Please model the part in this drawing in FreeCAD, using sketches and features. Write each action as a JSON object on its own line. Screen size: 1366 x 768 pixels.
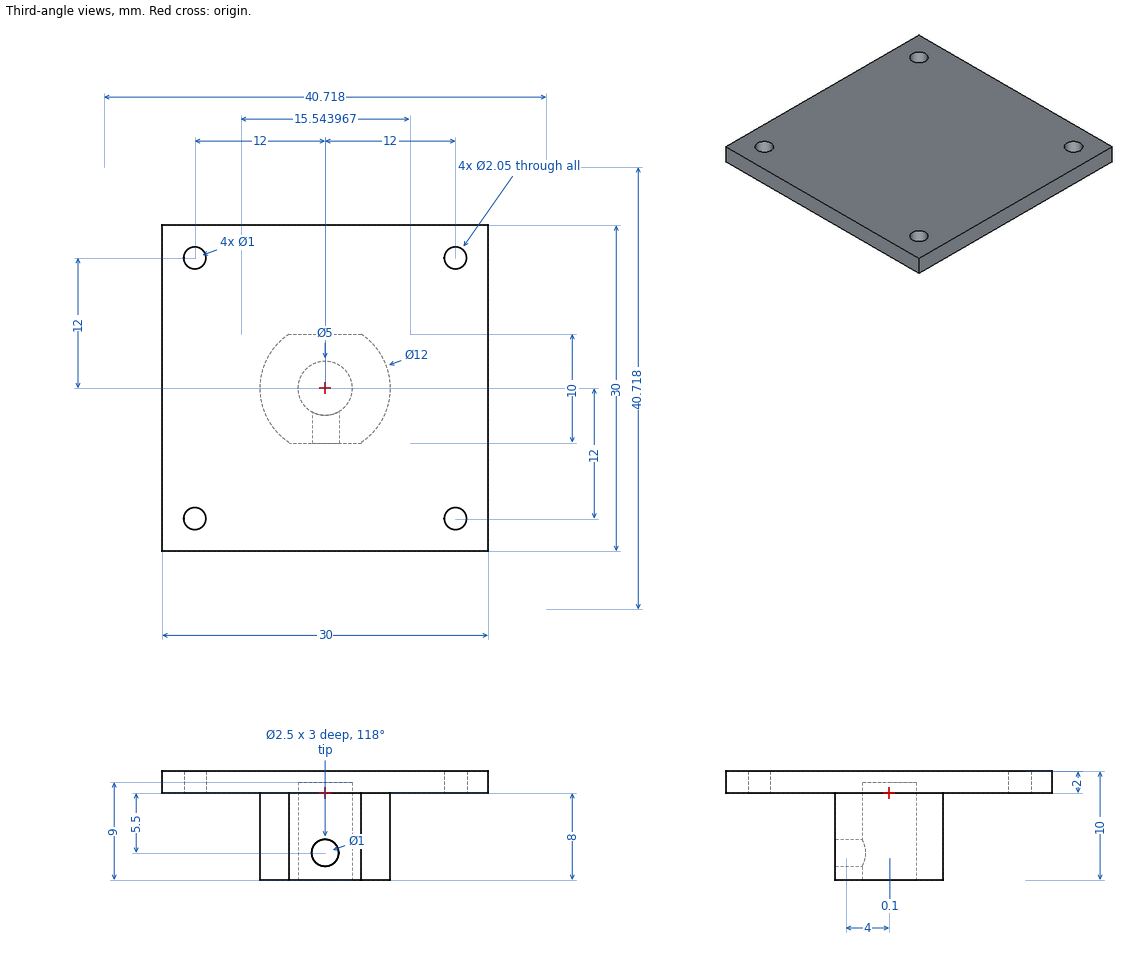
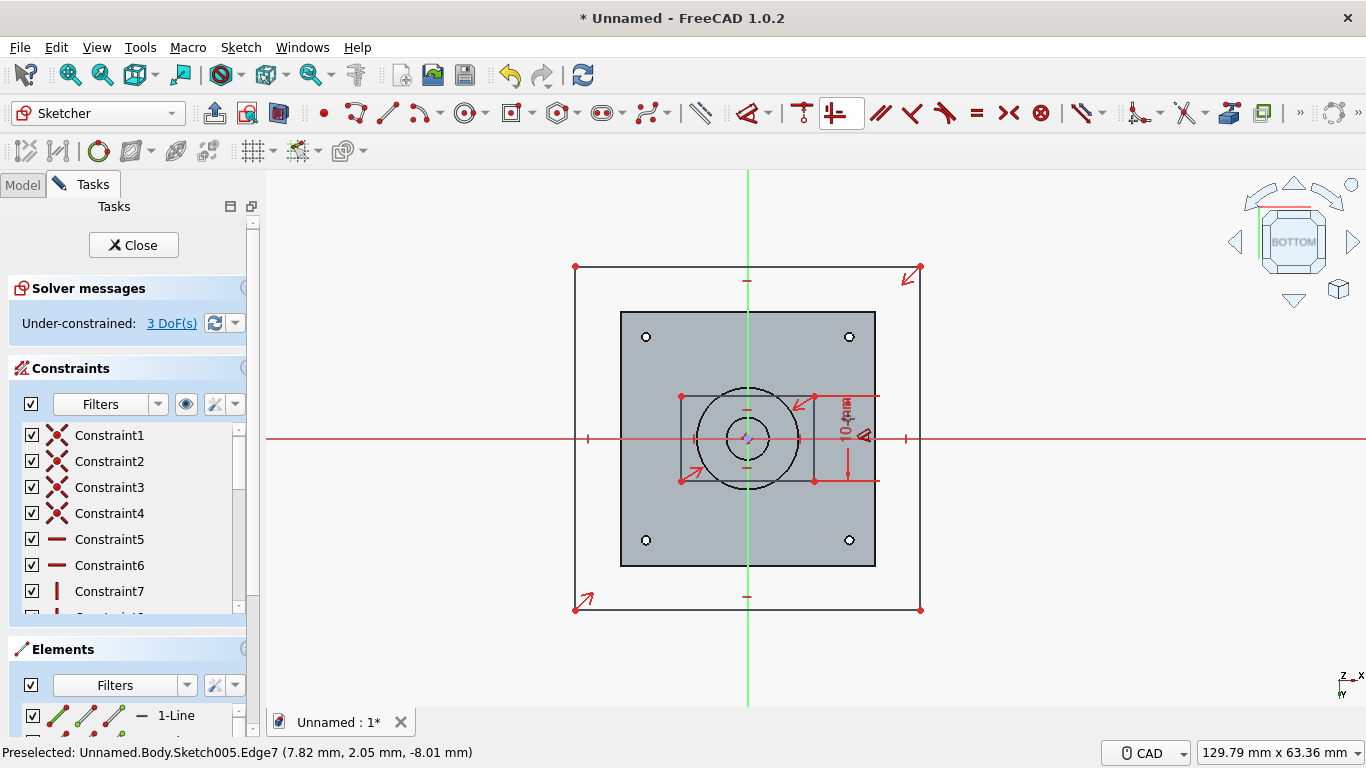
{"action": "left_click", "coordinate": [679, 610]}
{"action": "left_click", "coordinate": [668, 644]}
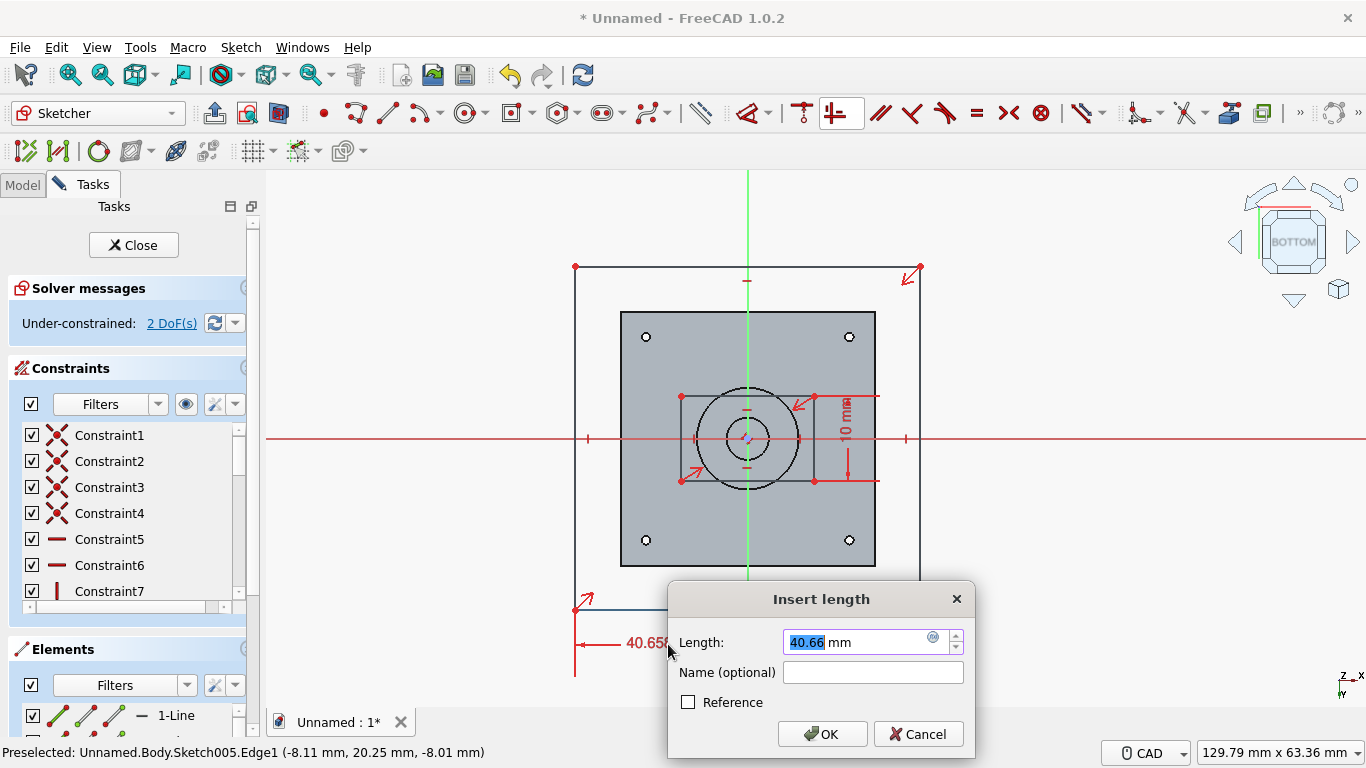
{"action": "type", "text": "40.718"}
{"action": "key", "text": "Return"}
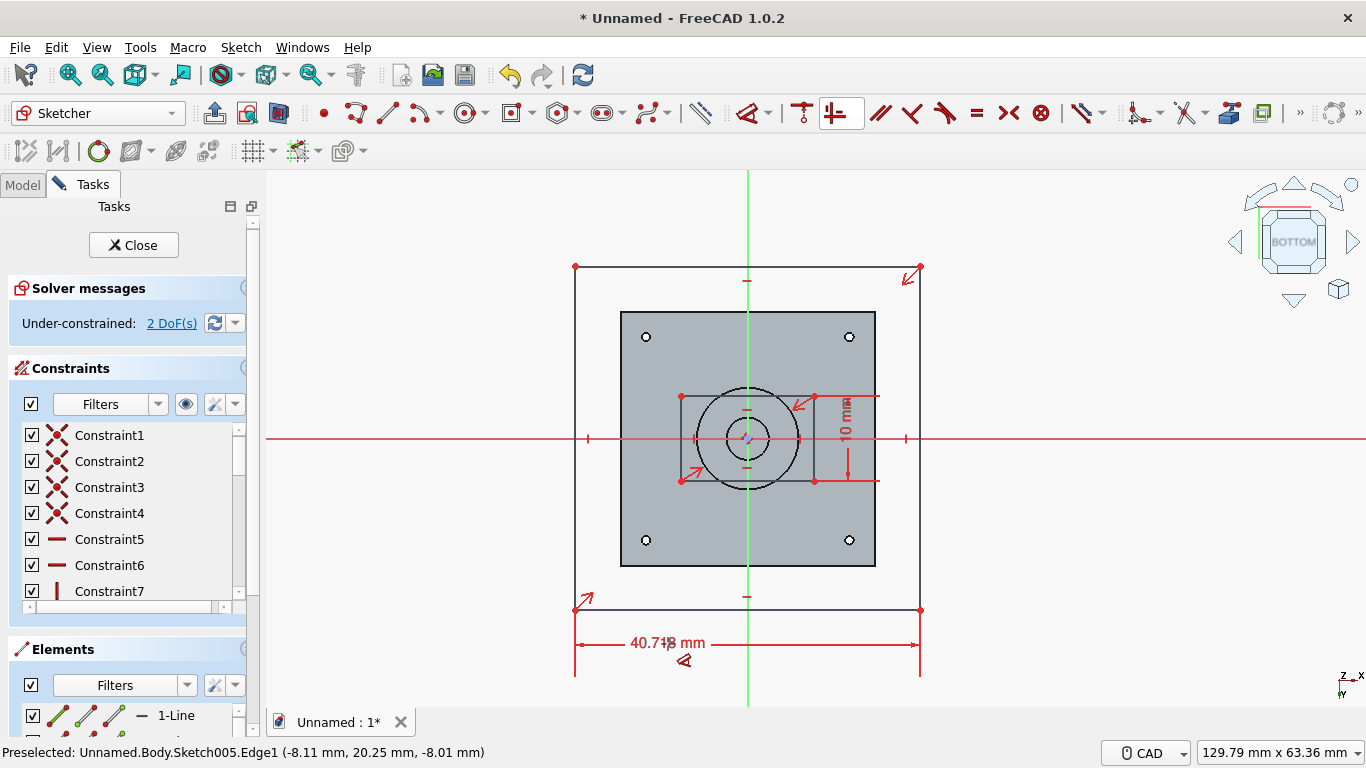
{"action": "left_click", "coordinate": [920, 507]}
{"action": "left_click", "coordinate": [954, 360]}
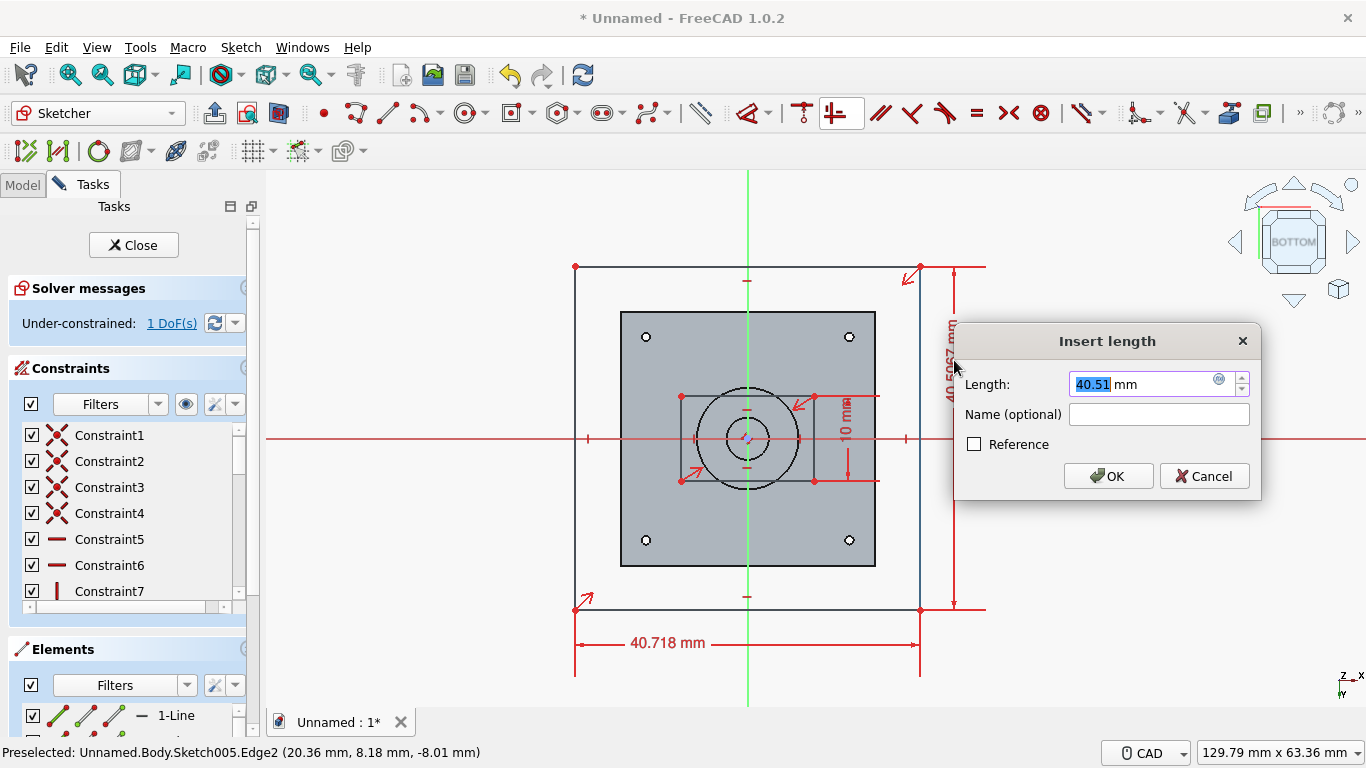
{"action": "type", "text": "40.718"}
{"action": "key", "text": "Return"}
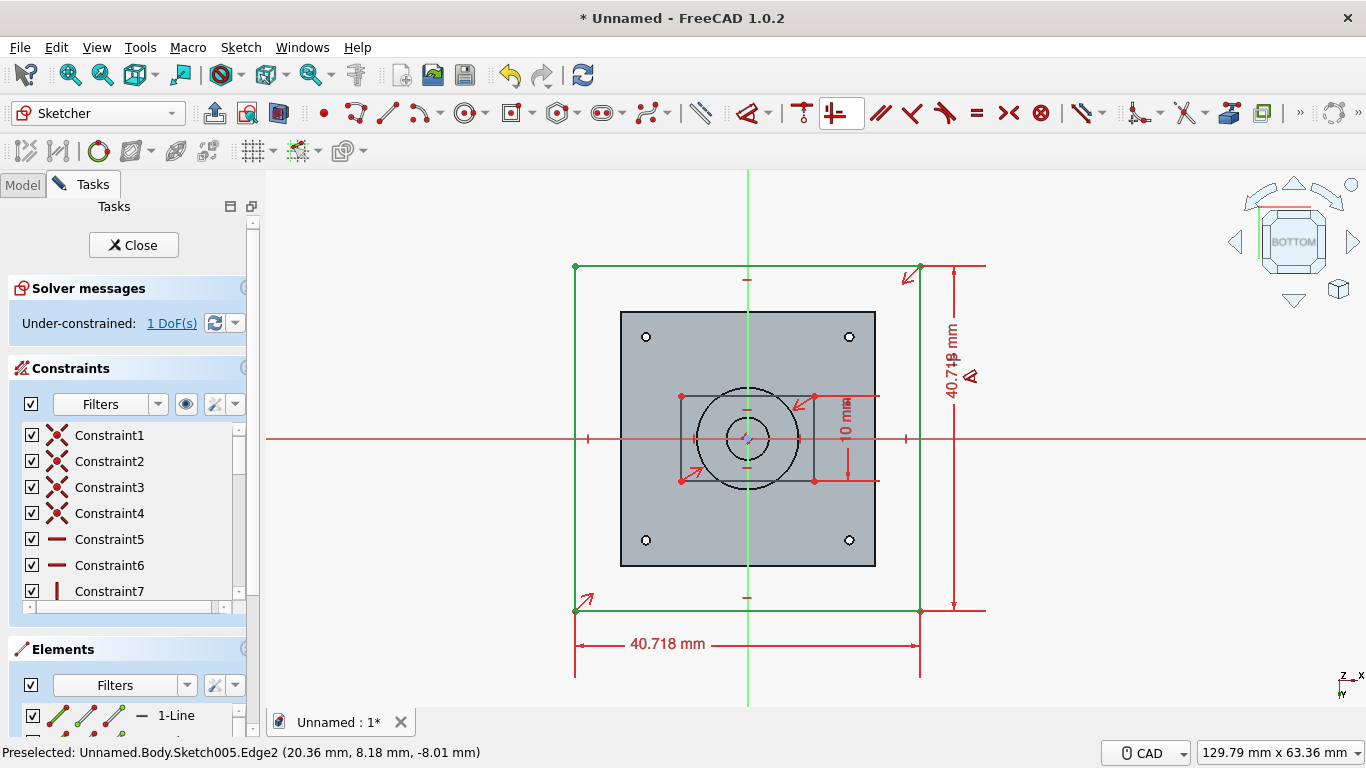
{"action": "left_click", "coordinate": [721, 481]}
{"action": "left_click", "coordinate": [717, 515]}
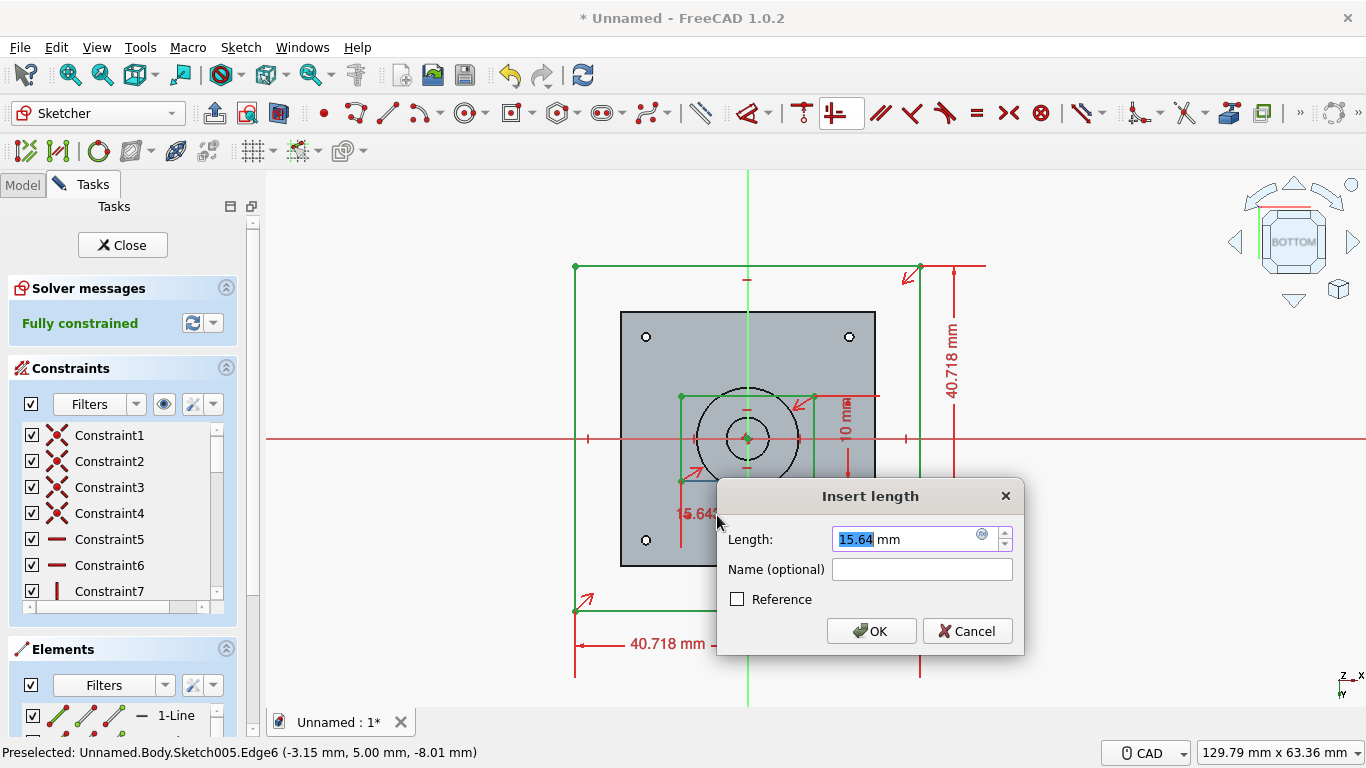
{"action": "type", "text": "15.543967"}
{"action": "key", "text": "Return"}
{"action": "key", "text": "Escape"}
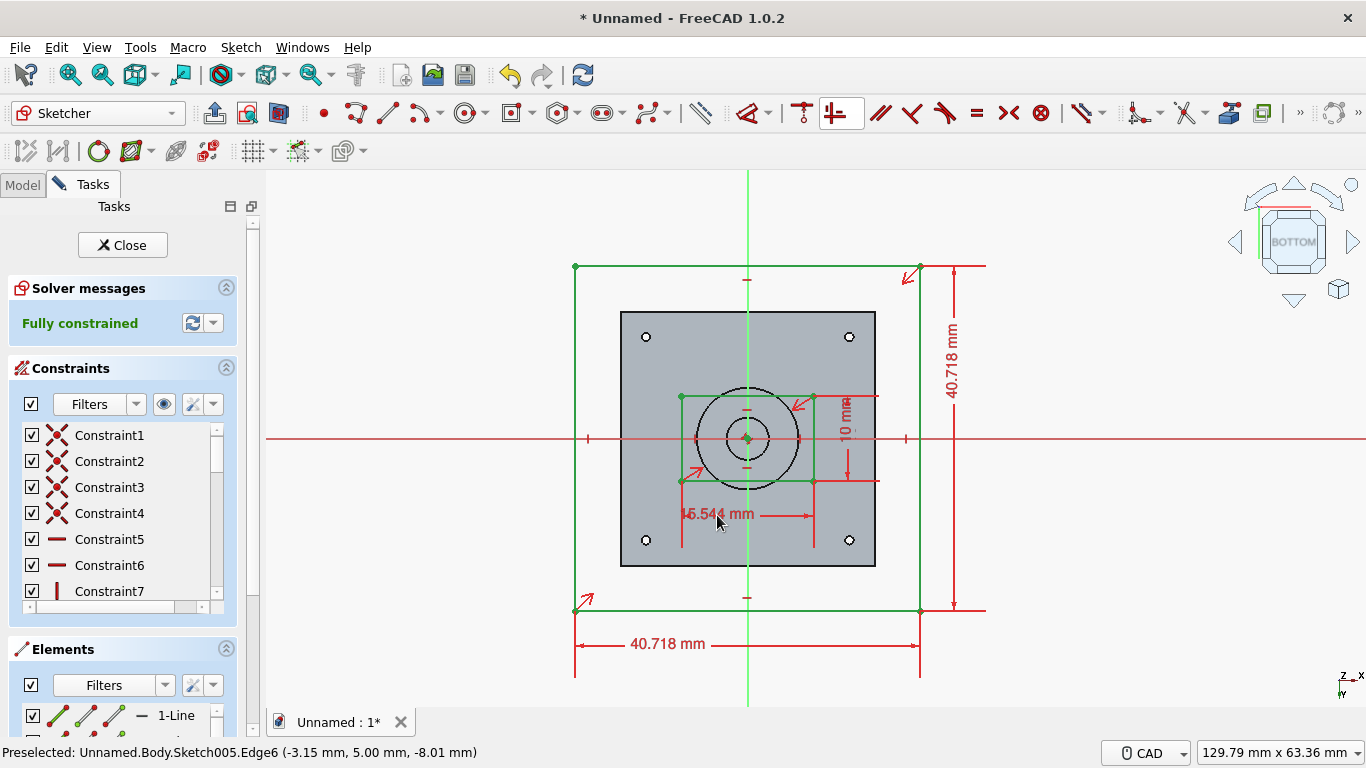
{"action": "left_click", "coordinate": [123, 245]}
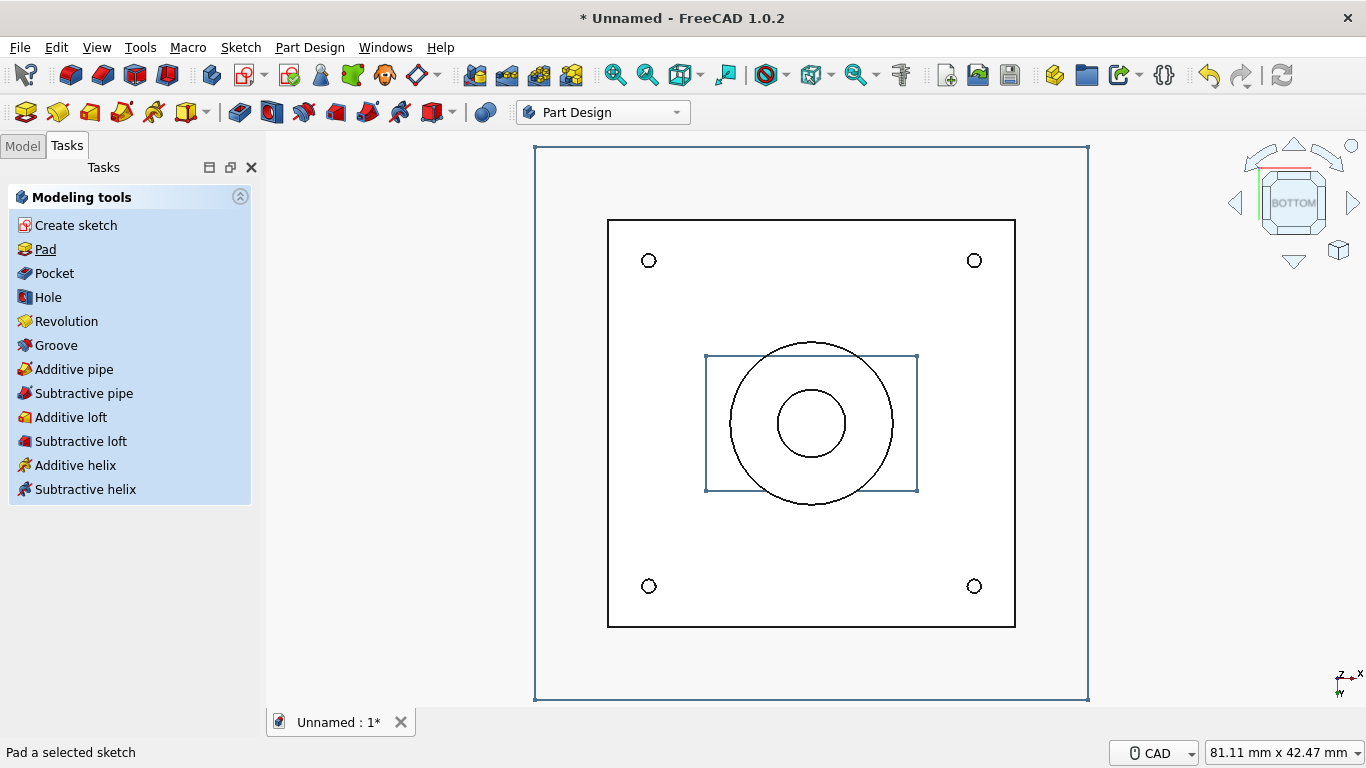
{"action": "left_click", "coordinate": [240, 112]}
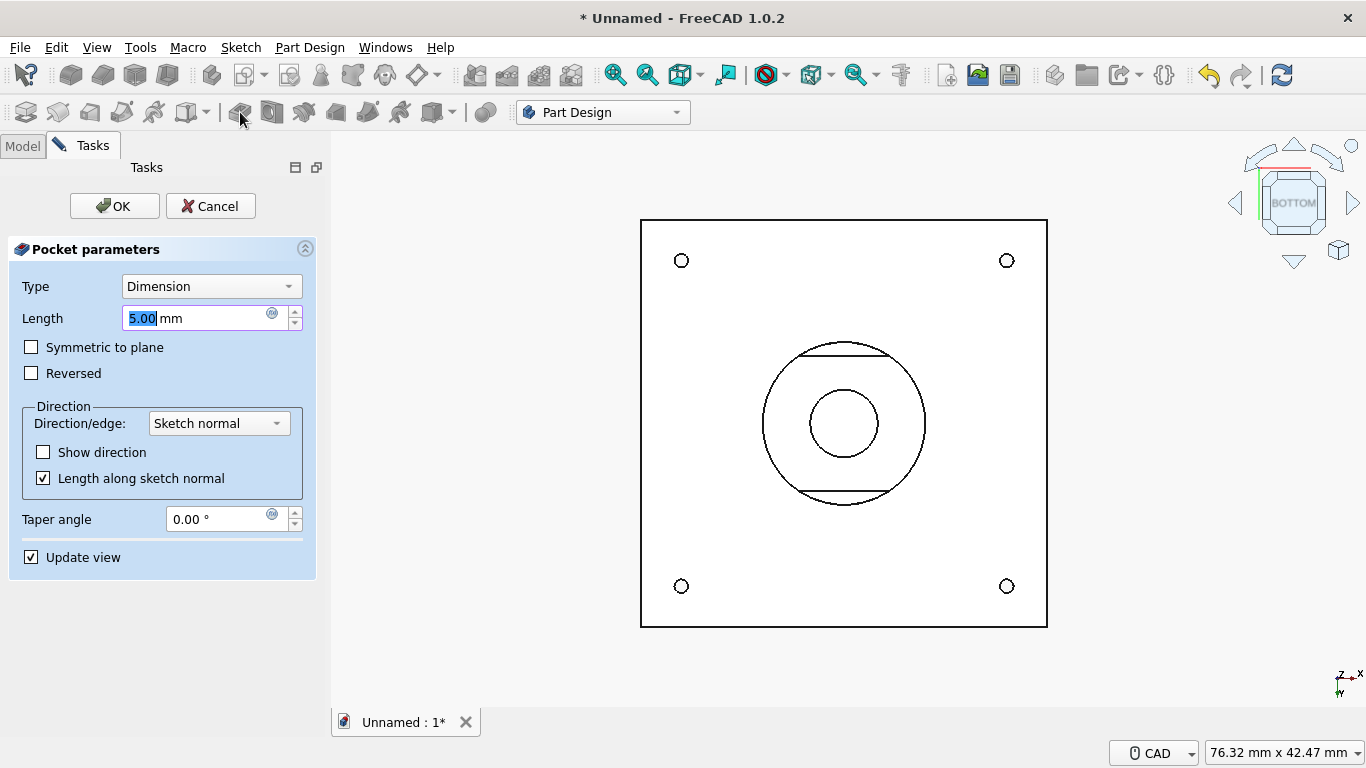
{"action": "type", "text": "8"}
{"action": "key", "text": "Tab"}